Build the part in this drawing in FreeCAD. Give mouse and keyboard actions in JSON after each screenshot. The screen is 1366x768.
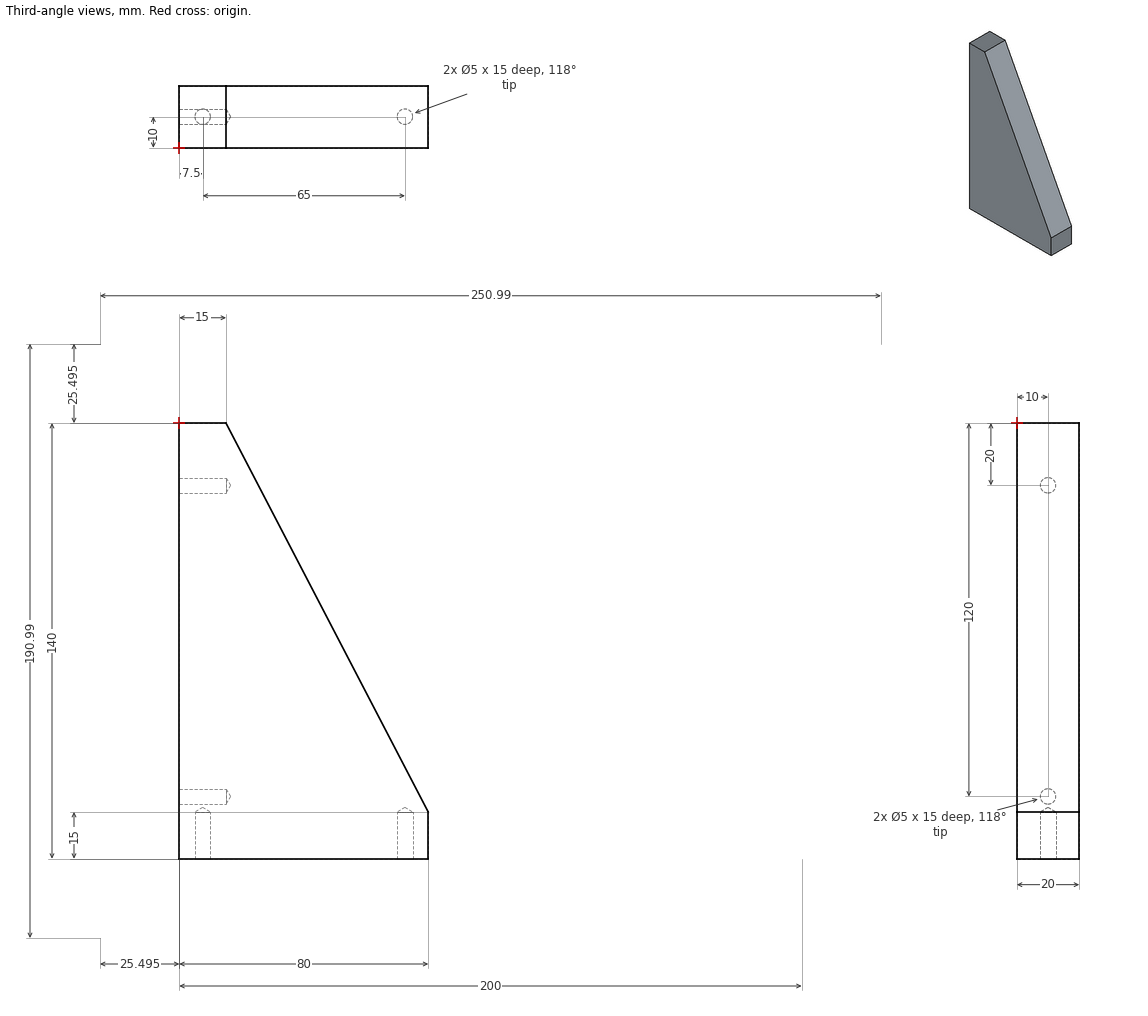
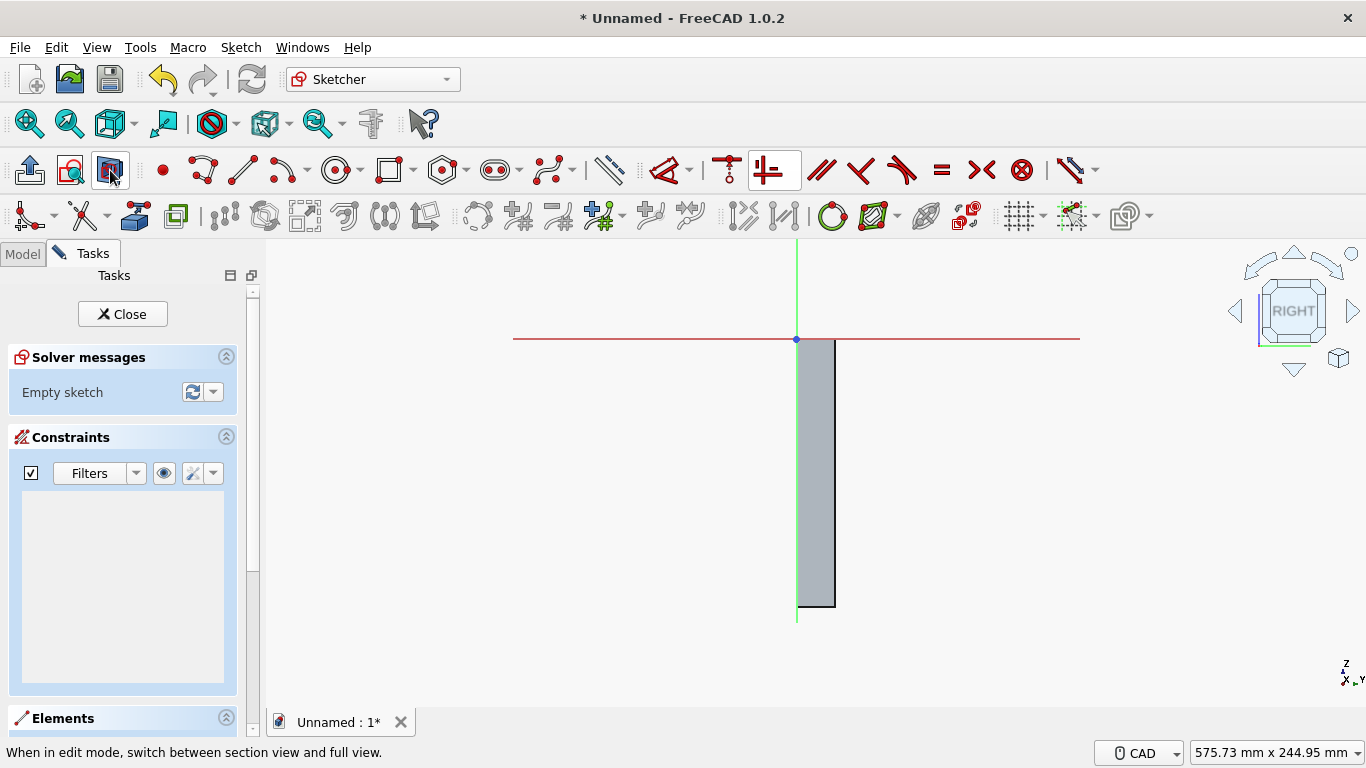
{"action": "key", "text": "g c"}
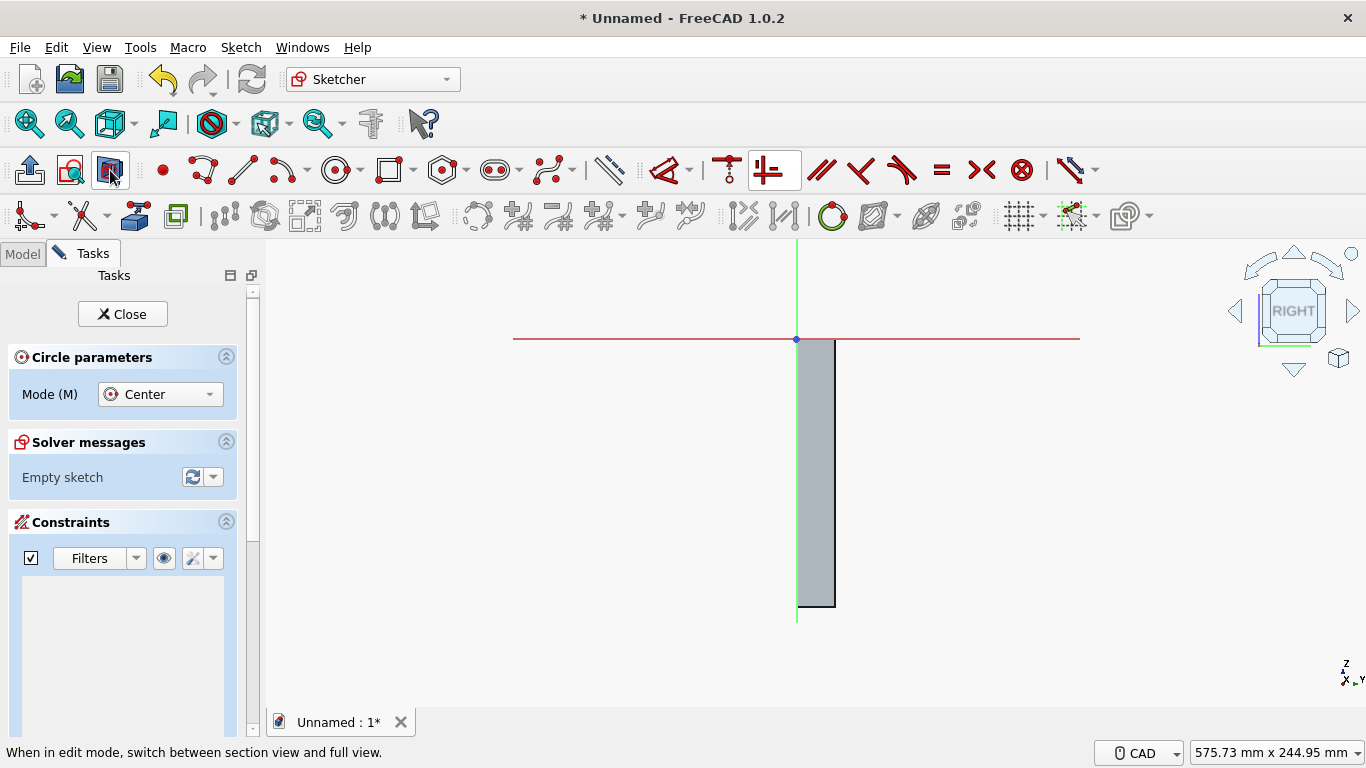
{"action": "scroll", "coordinate": [816, 569], "scroll_direction": "up", "scroll_amount": 8}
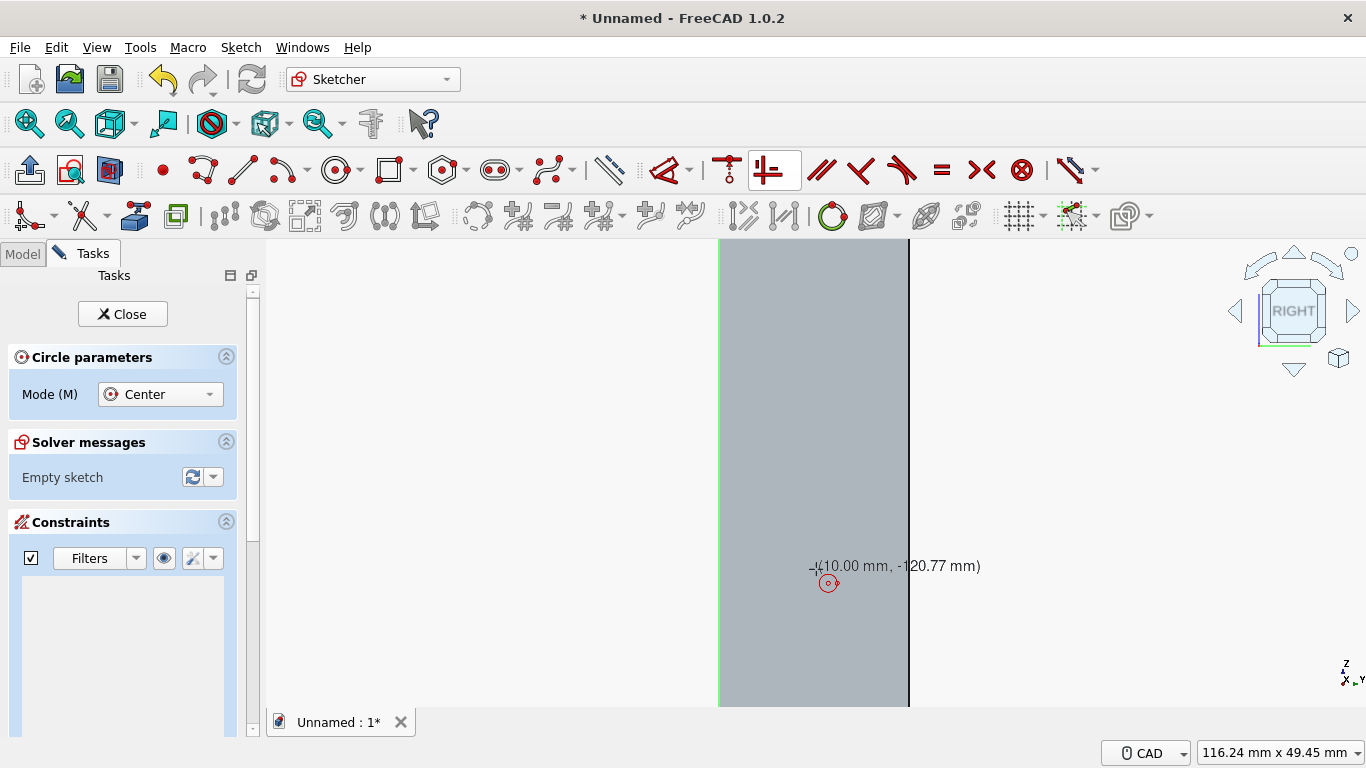
{"action": "scroll", "coordinate": [737, 625], "scroll_direction": "down", "scroll_amount": 7}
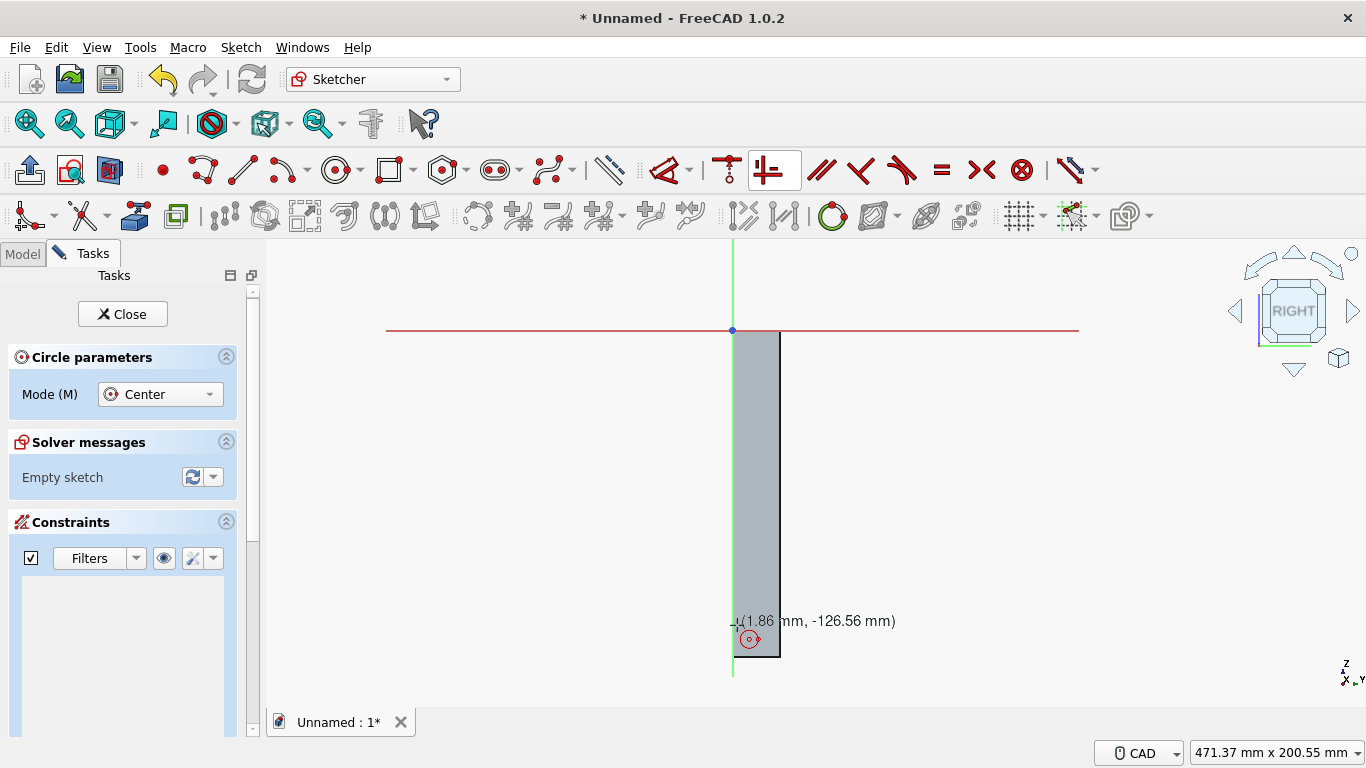
{"action": "left_click", "coordinate": [756, 611]}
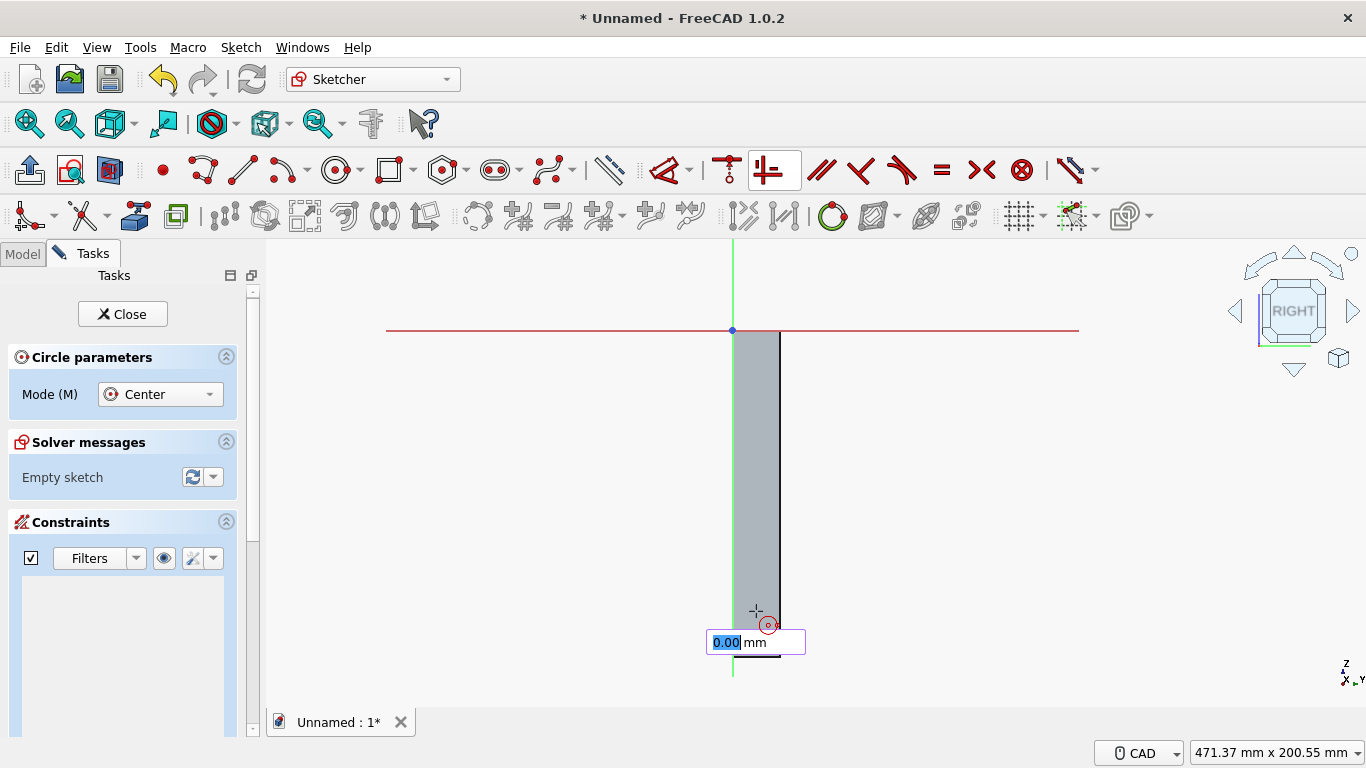
{"action": "scroll", "coordinate": [760, 606], "scroll_direction": "up", "scroll_amount": 6}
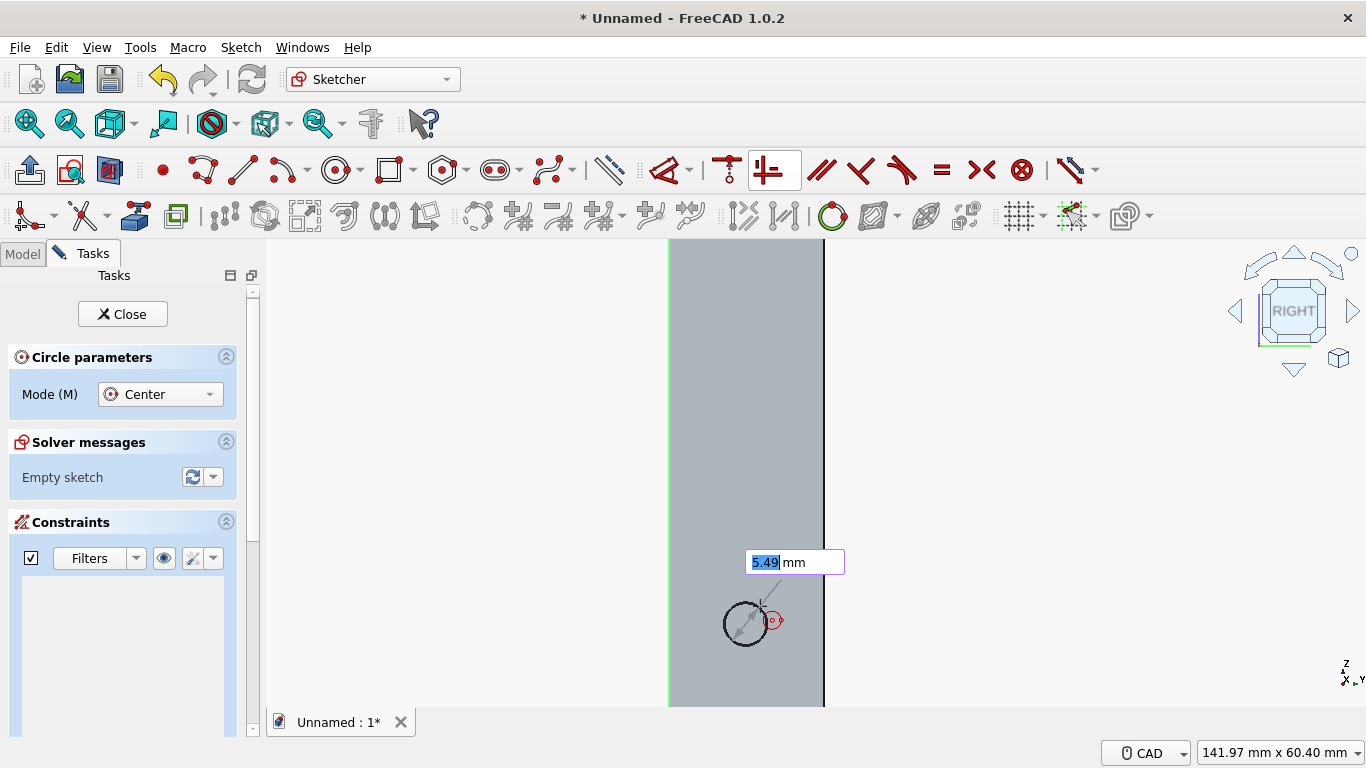
{"action": "left_click", "coordinate": [760, 606]}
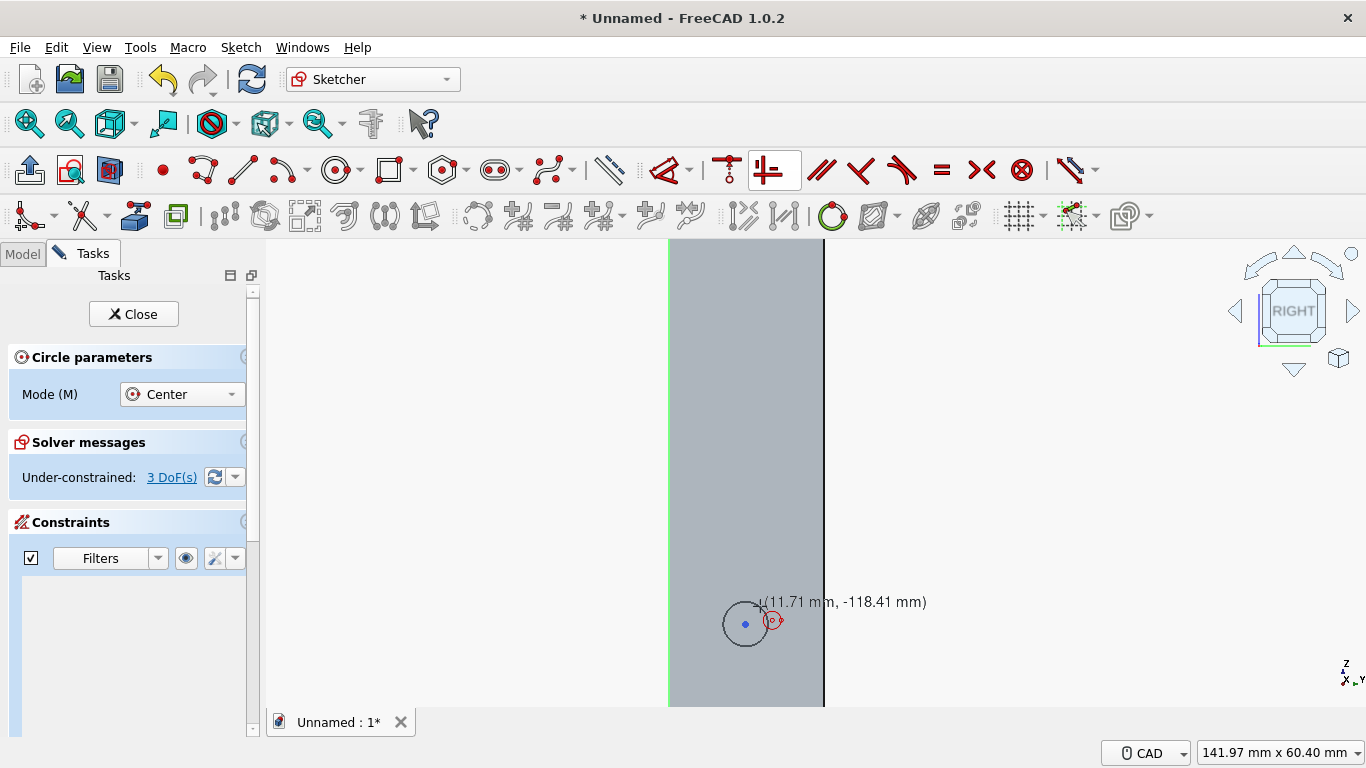
{"action": "scroll", "coordinate": [760, 606], "scroll_direction": "down", "scroll_amount": 6}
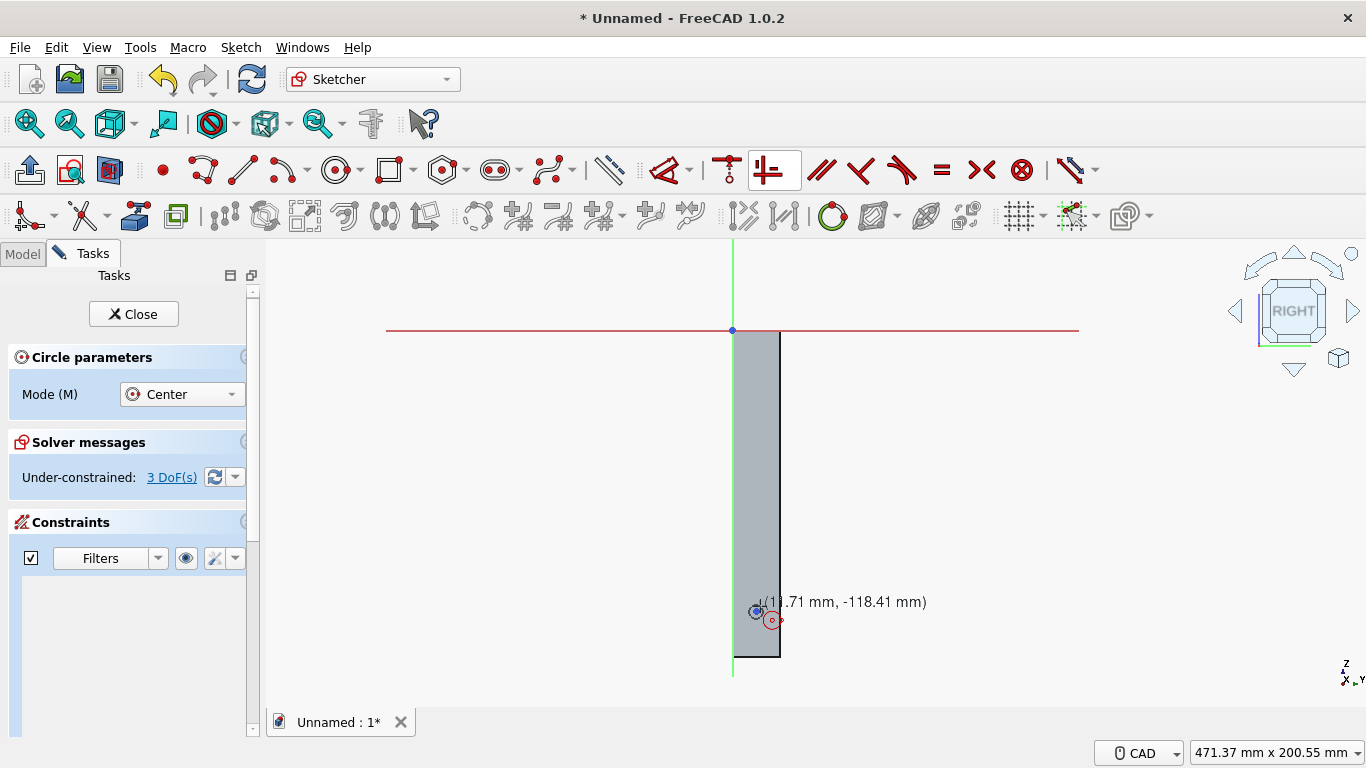
{"action": "scroll", "coordinate": [756, 377], "scroll_direction": "up", "scroll_amount": 7}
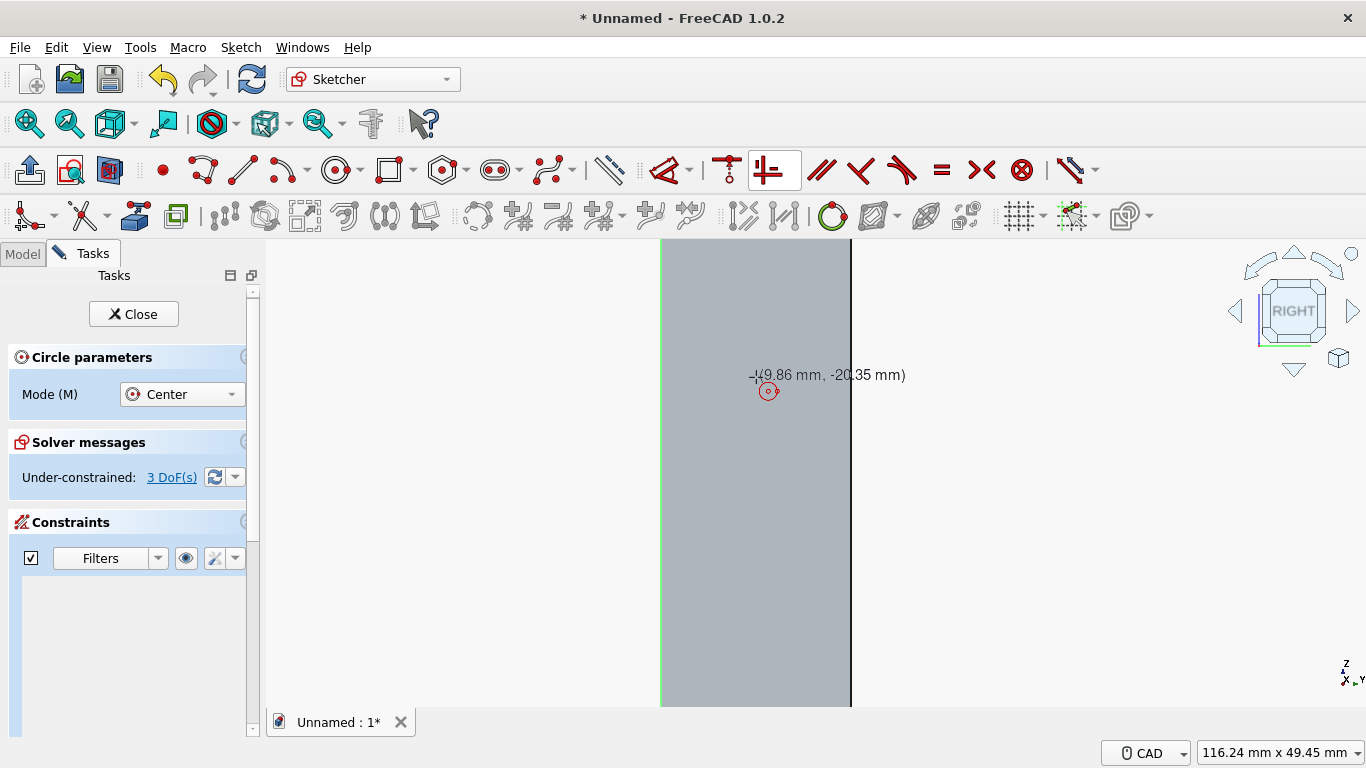
{"action": "scroll", "coordinate": [756, 377], "scroll_direction": "down", "scroll_amount": 7}